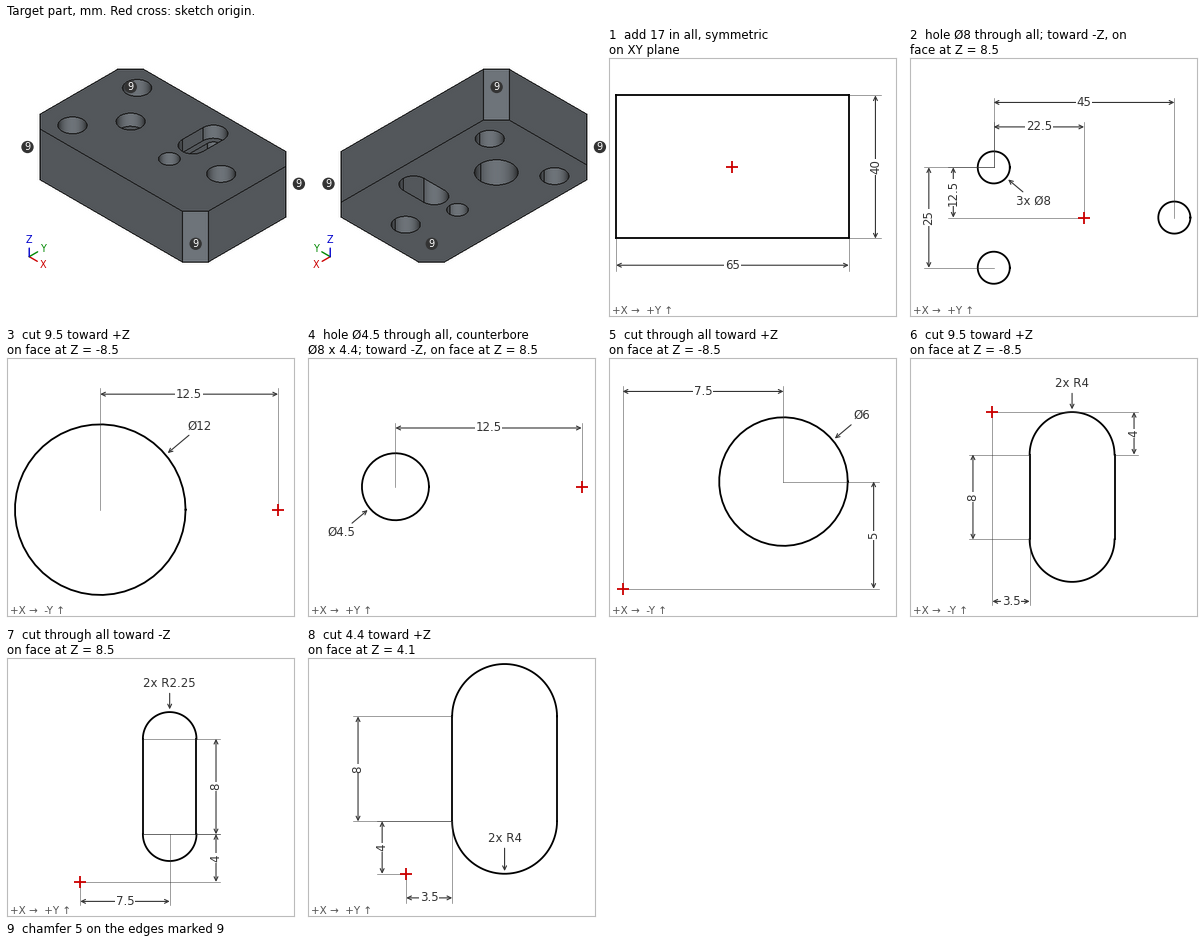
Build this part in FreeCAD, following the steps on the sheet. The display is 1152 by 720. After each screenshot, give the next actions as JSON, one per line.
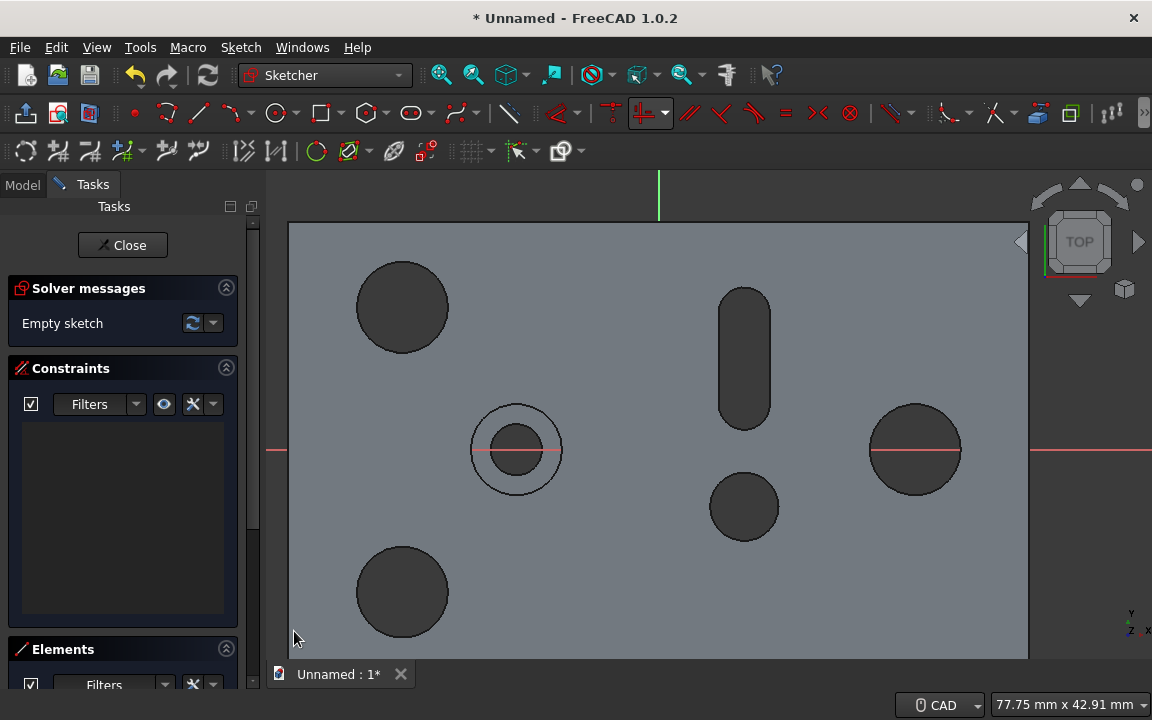
{"action": "scroll", "coordinate": [826, 291], "scroll_direction": "up", "scroll_amount": 3}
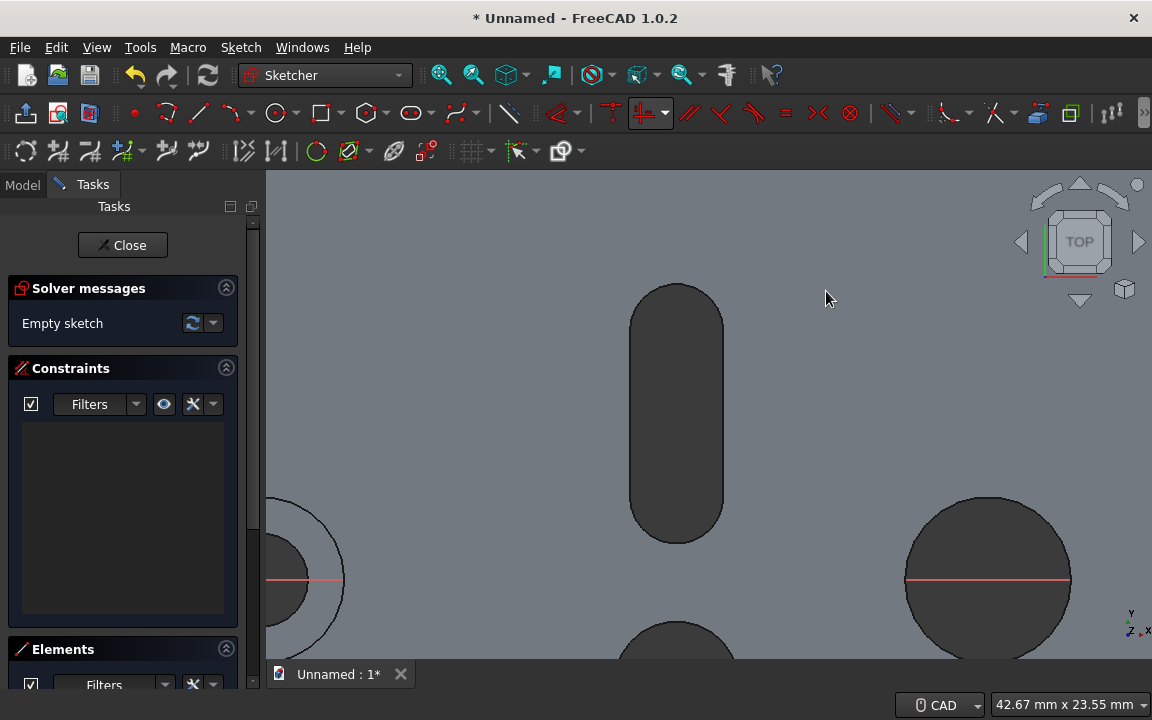
{"action": "left_click", "coordinate": [412, 114]}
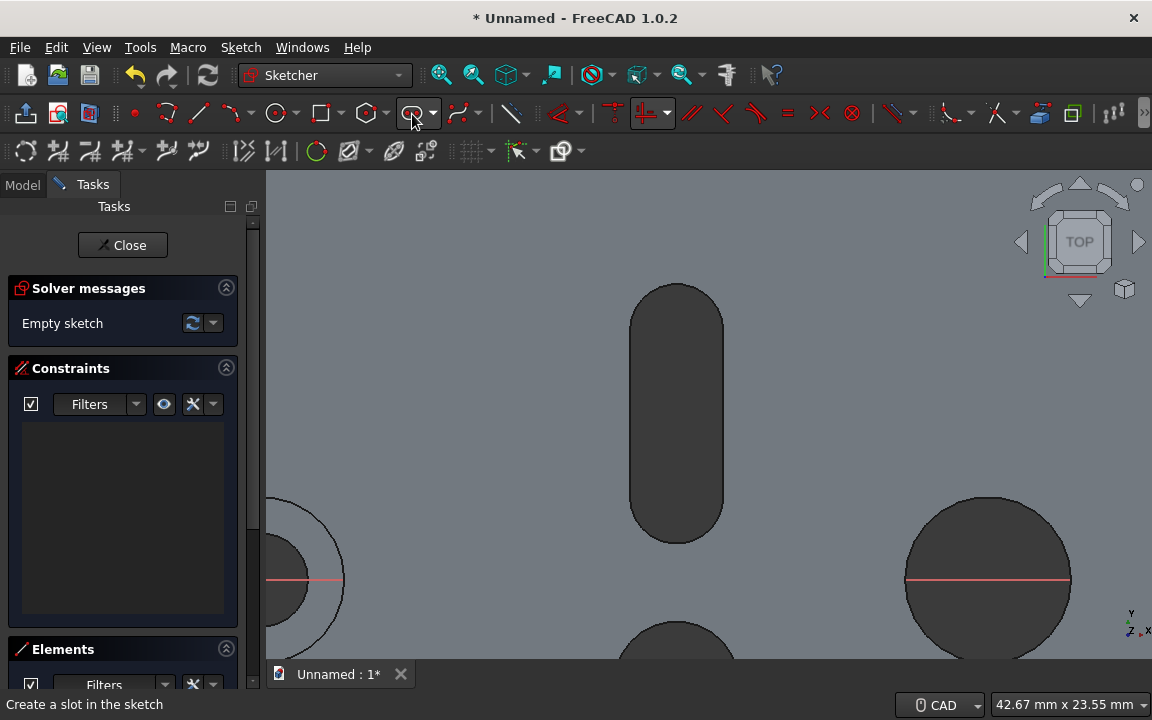
{"action": "left_click", "coordinate": [677, 497]}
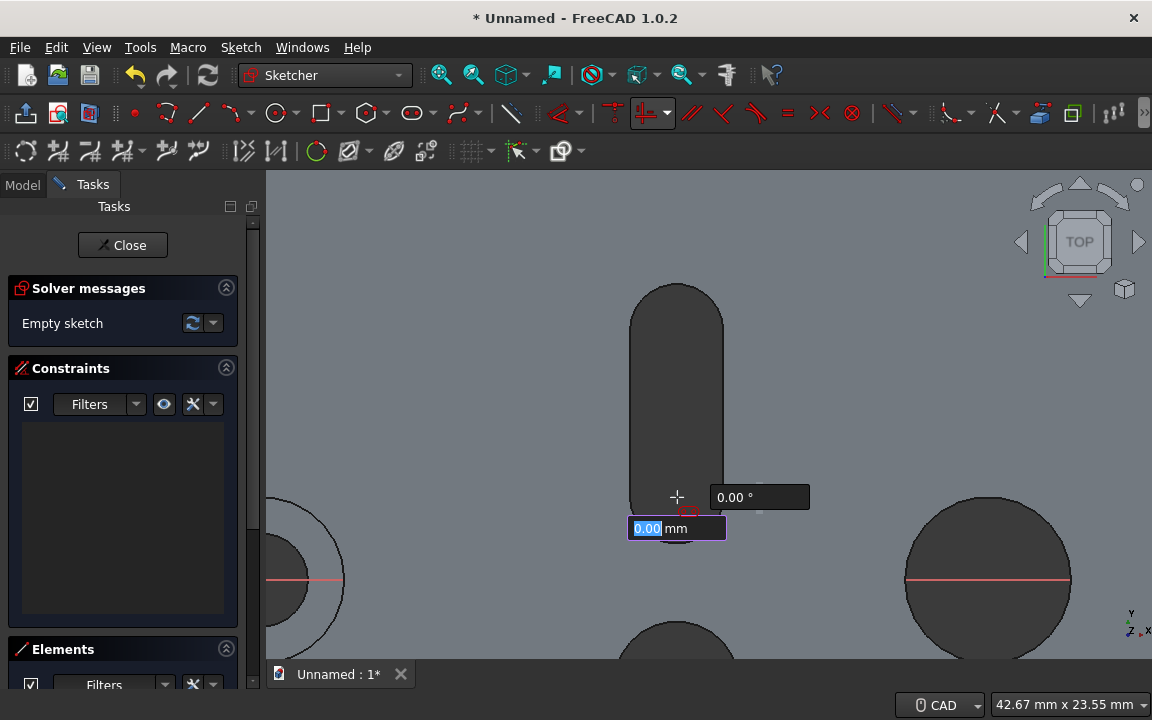
{"action": "left_click", "coordinate": [677, 331]}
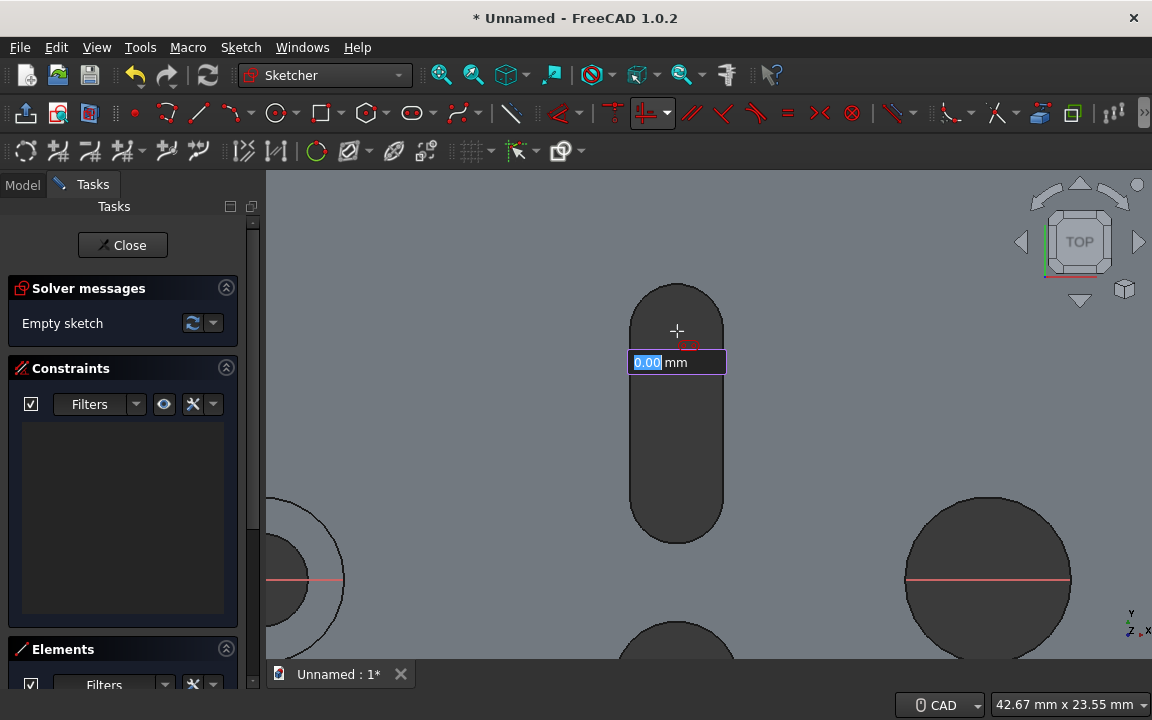
{"action": "left_click", "coordinate": [594, 414]}
{"action": "key", "text": "Escape"}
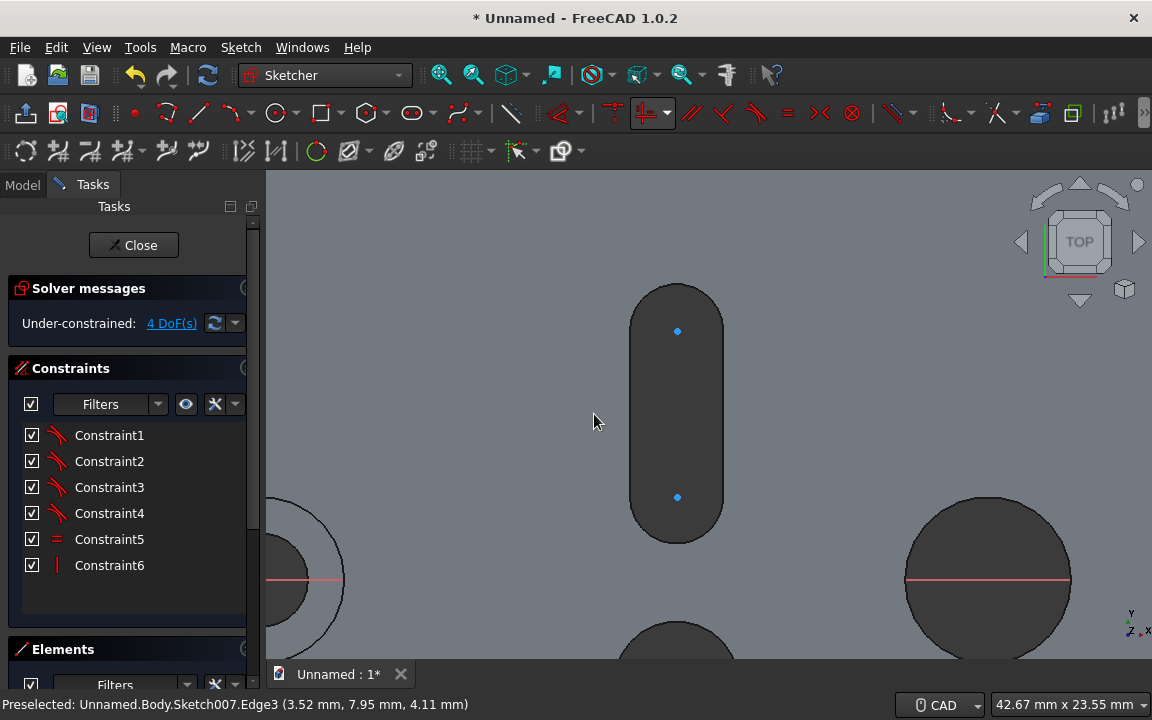
{"action": "key", "text": "d"}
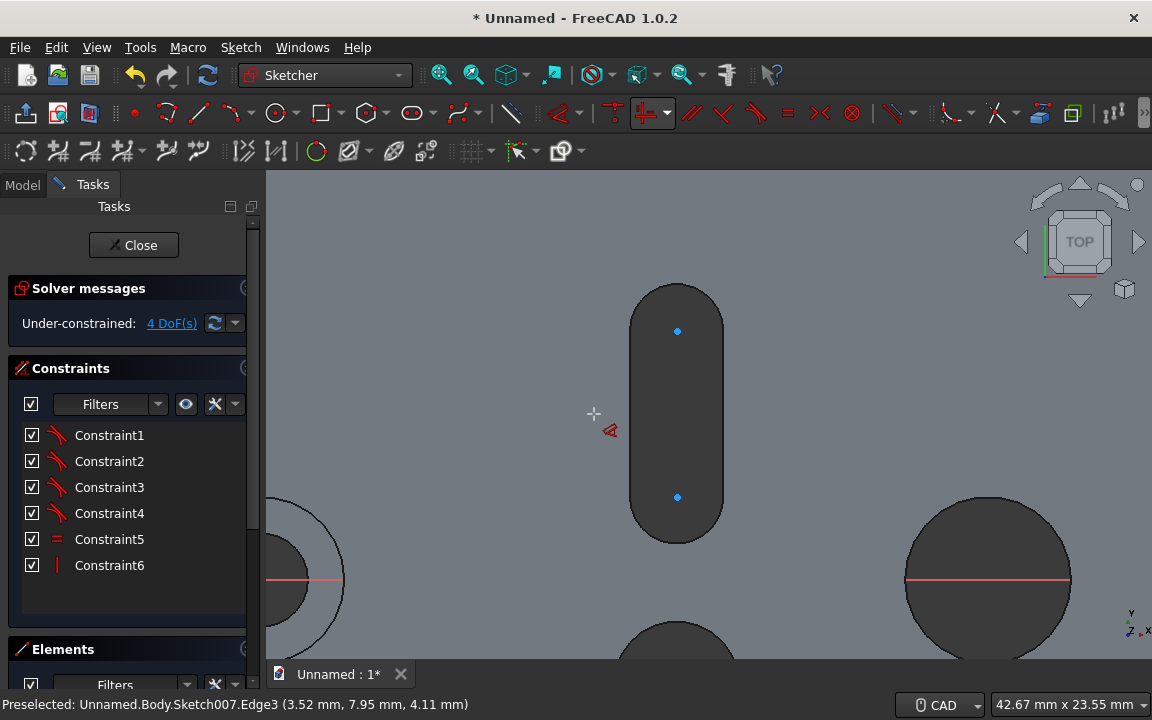
{"action": "left_click", "coordinate": [628, 565]}
{"action": "left_click", "coordinate": [573, 547]}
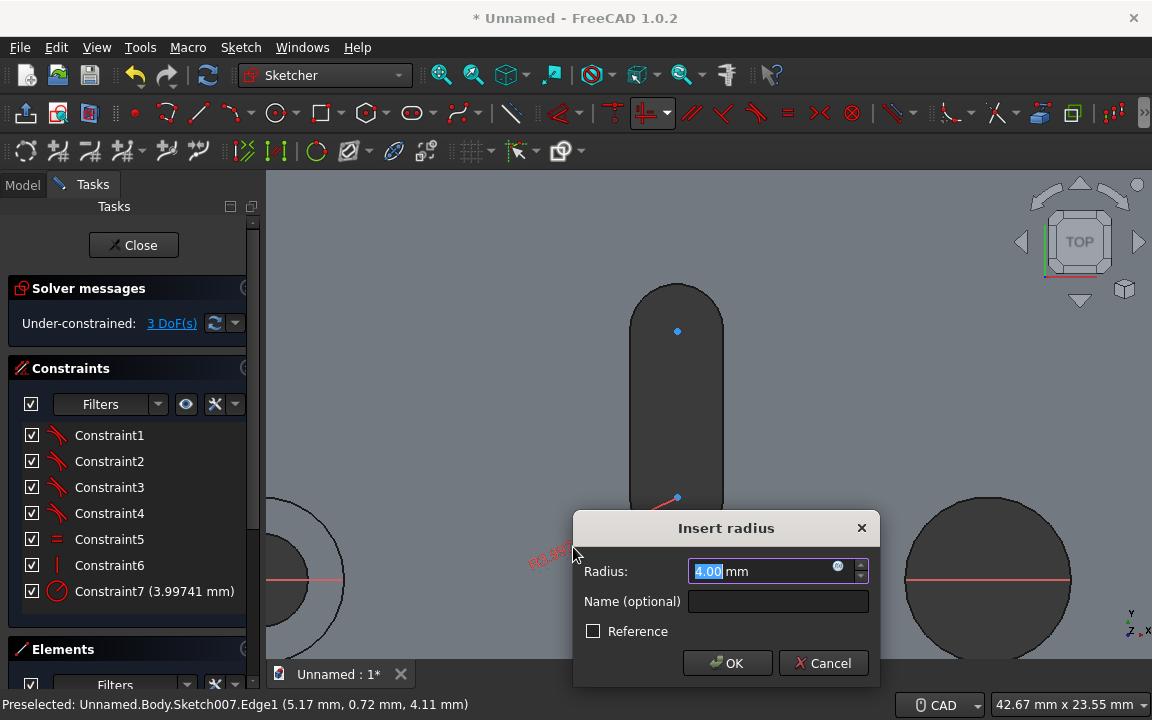
{"action": "type", "text": "4"}
{"action": "key", "text": "Return"}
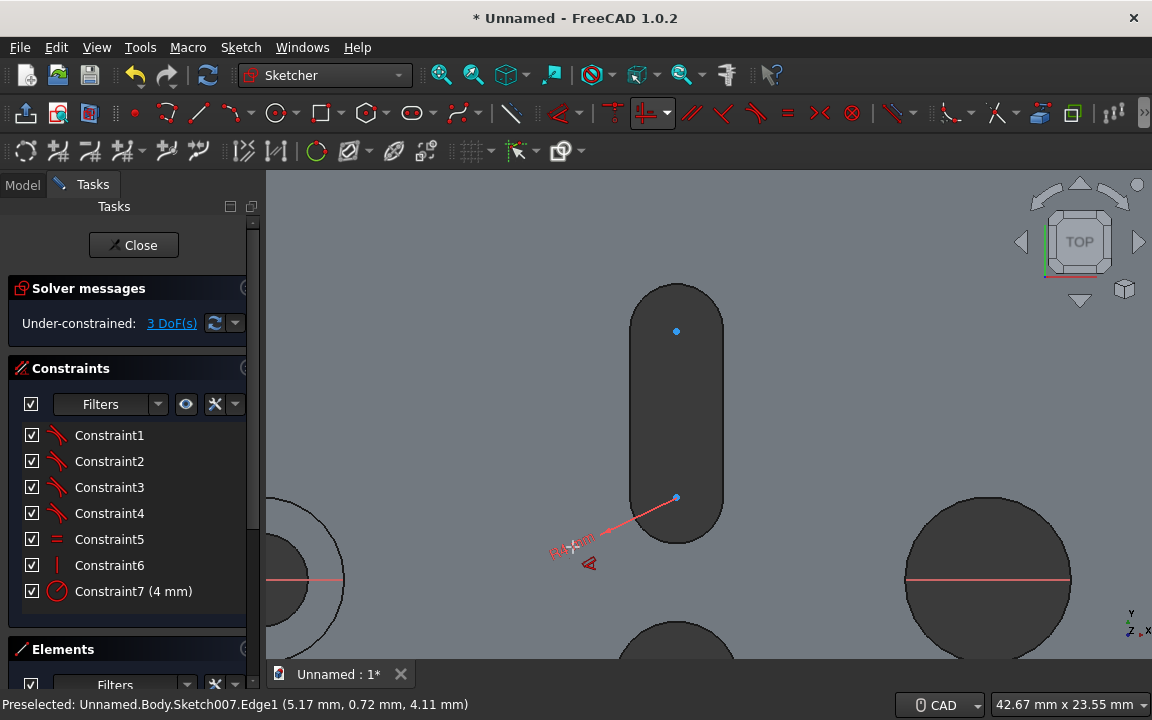
{"action": "left_click", "coordinate": [594, 448]}
{"action": "left_click", "coordinate": [560, 415]}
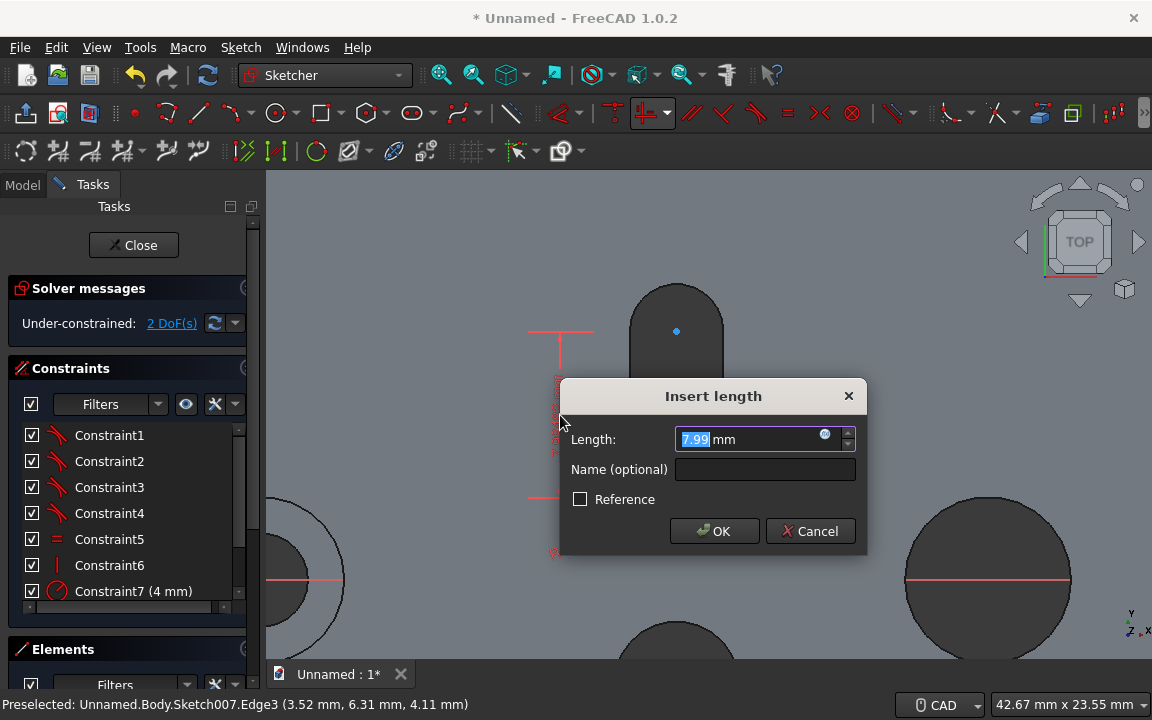
{"action": "type", "text": "8"}
{"action": "key", "text": "Return"}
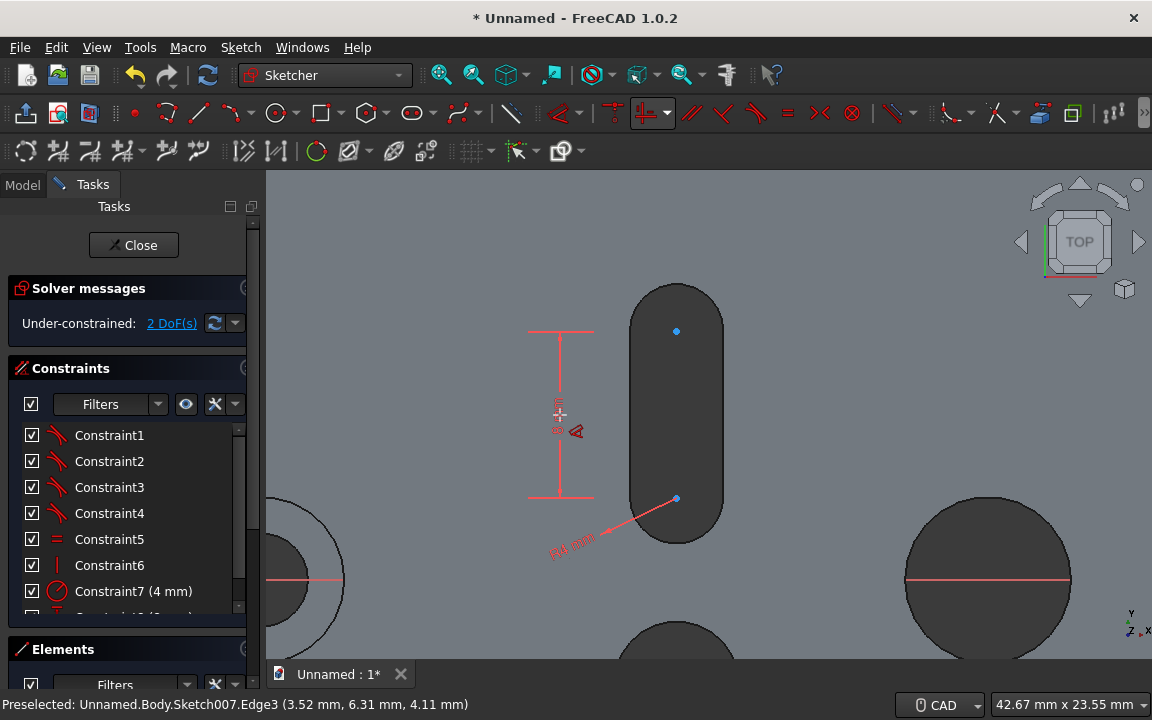
{"action": "left_click", "coordinate": [594, 498]}
{"action": "left_click", "coordinate": [487, 539]}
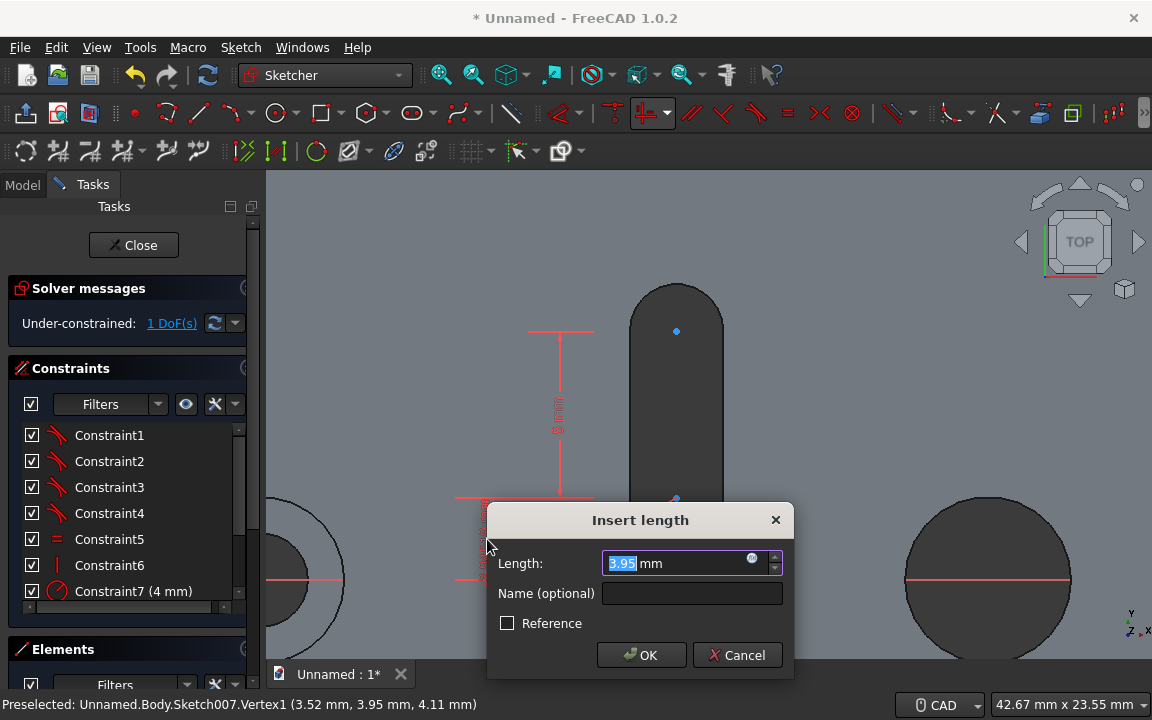
{"action": "type", "text": "4"}
{"action": "key", "text": "Return"}